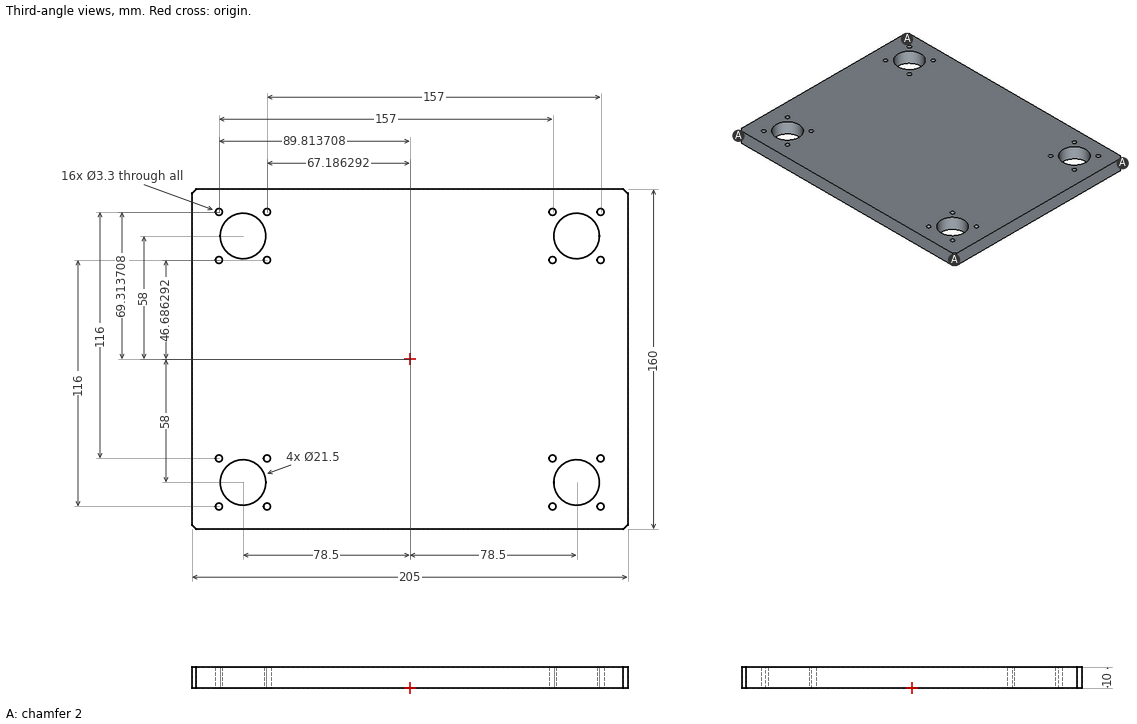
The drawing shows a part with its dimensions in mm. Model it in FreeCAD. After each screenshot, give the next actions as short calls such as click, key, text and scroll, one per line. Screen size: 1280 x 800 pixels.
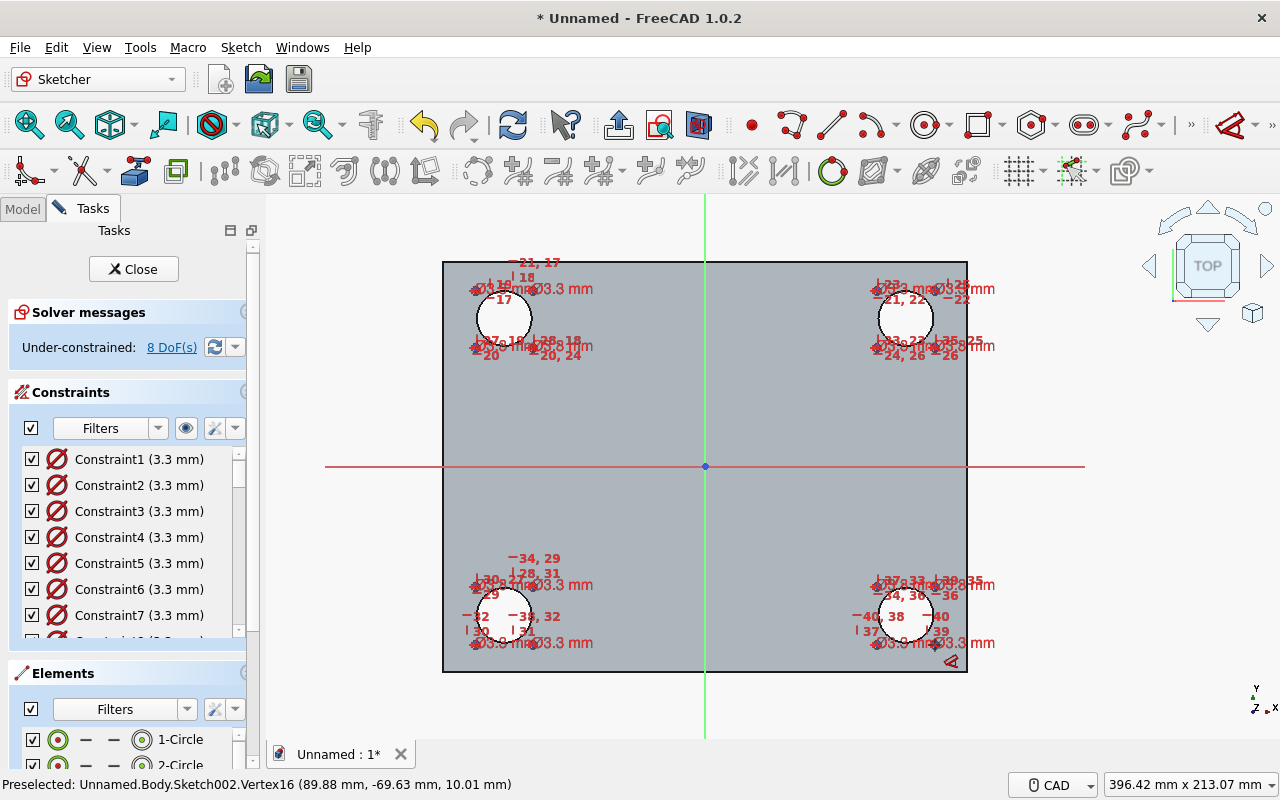
click(476, 291)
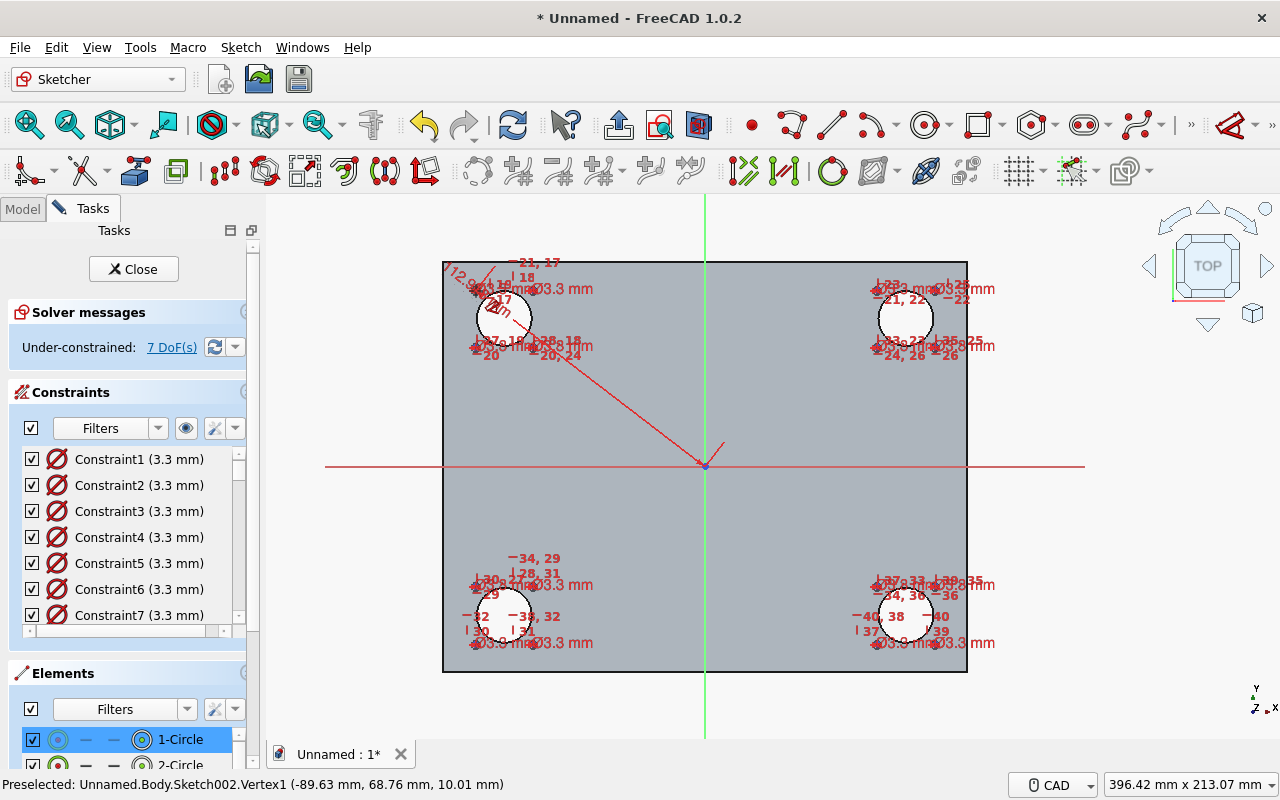
click(877, 291)
click(676, 257)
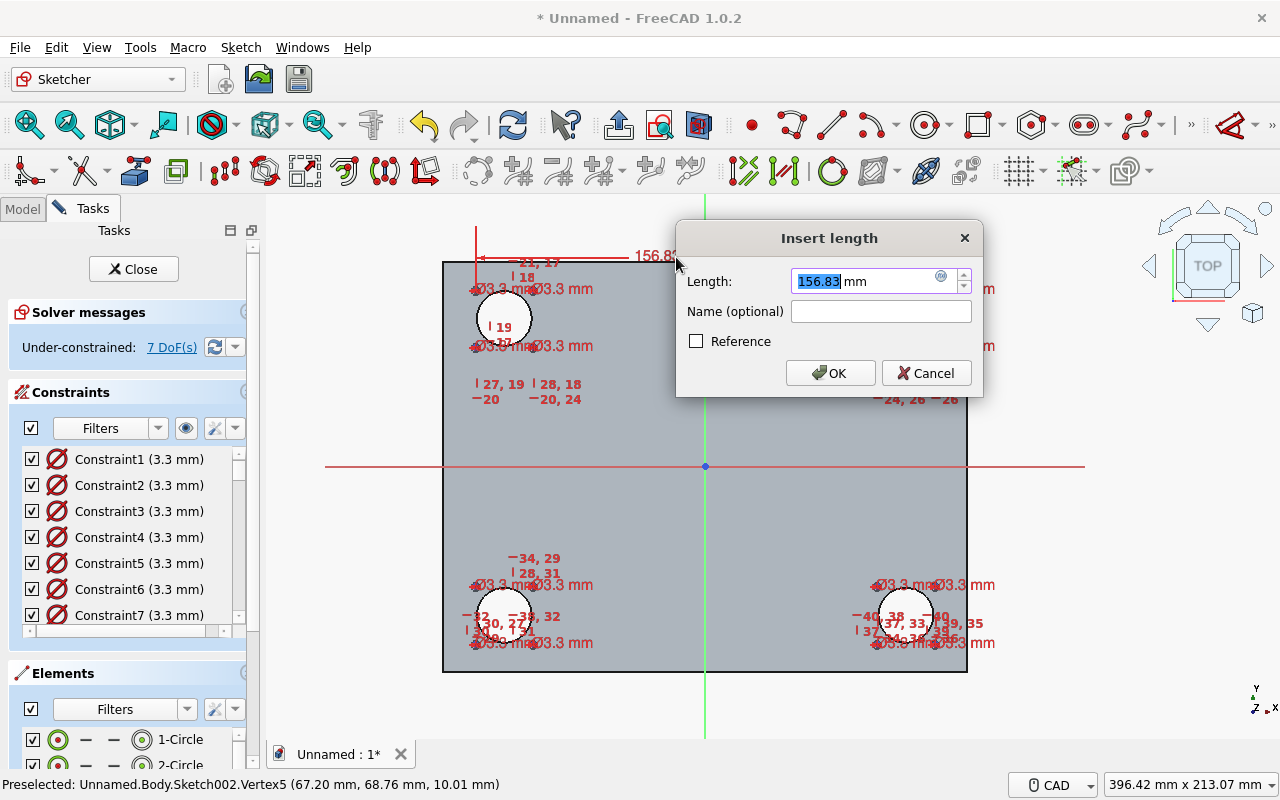
text(157)
key(Return)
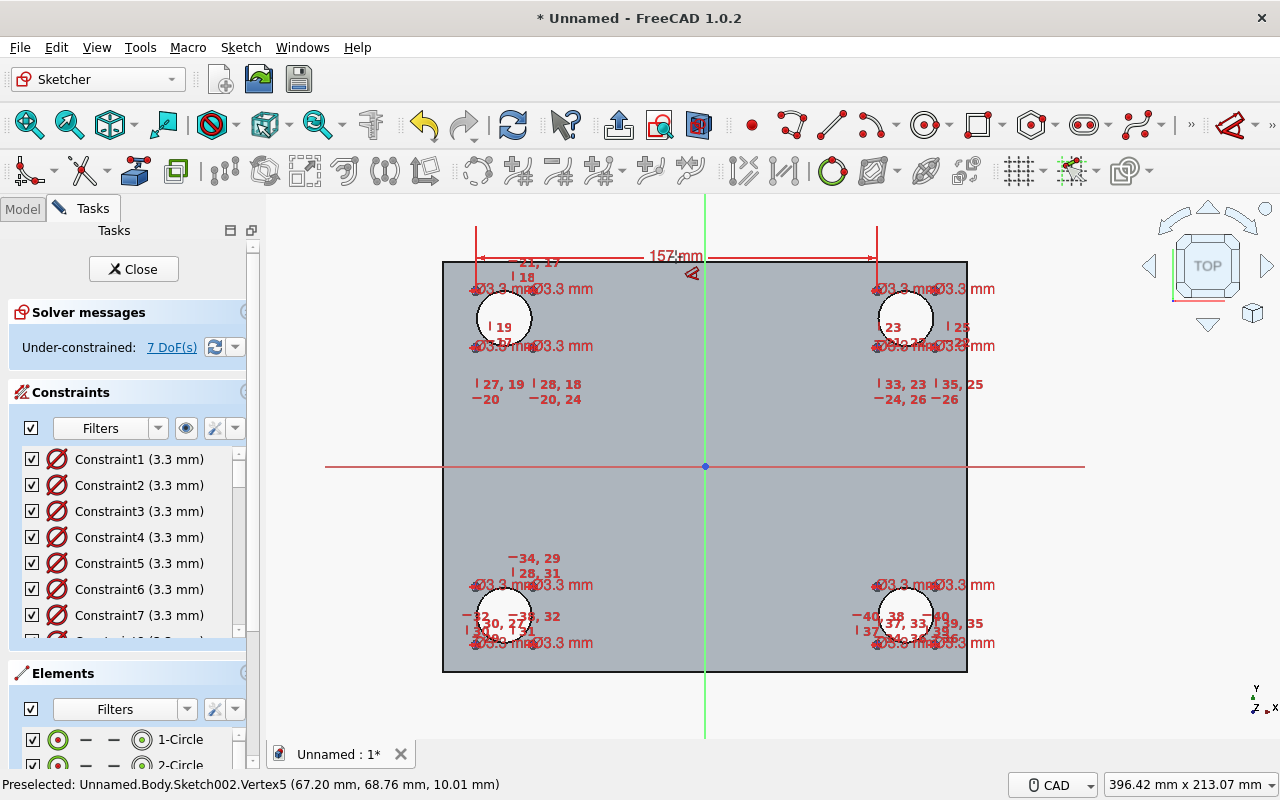
click(533, 291)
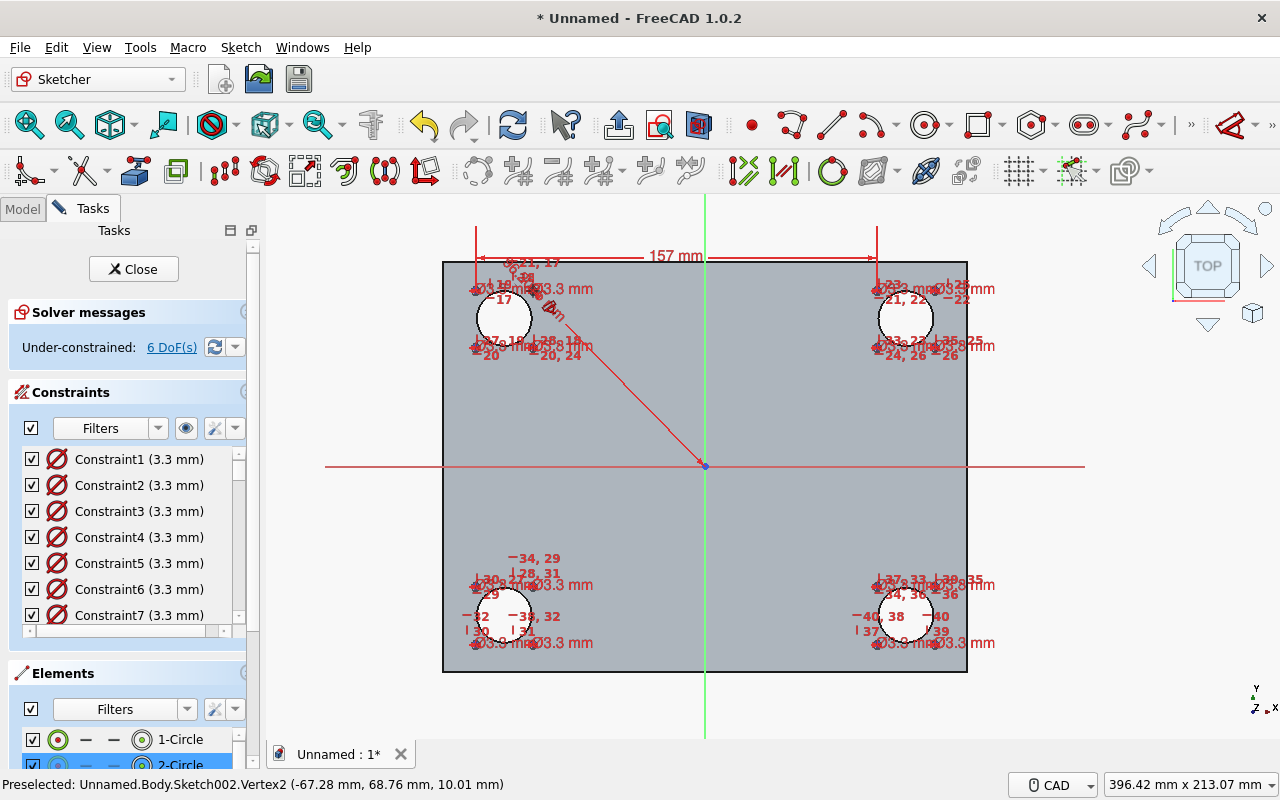
click(935, 291)
click(826, 257)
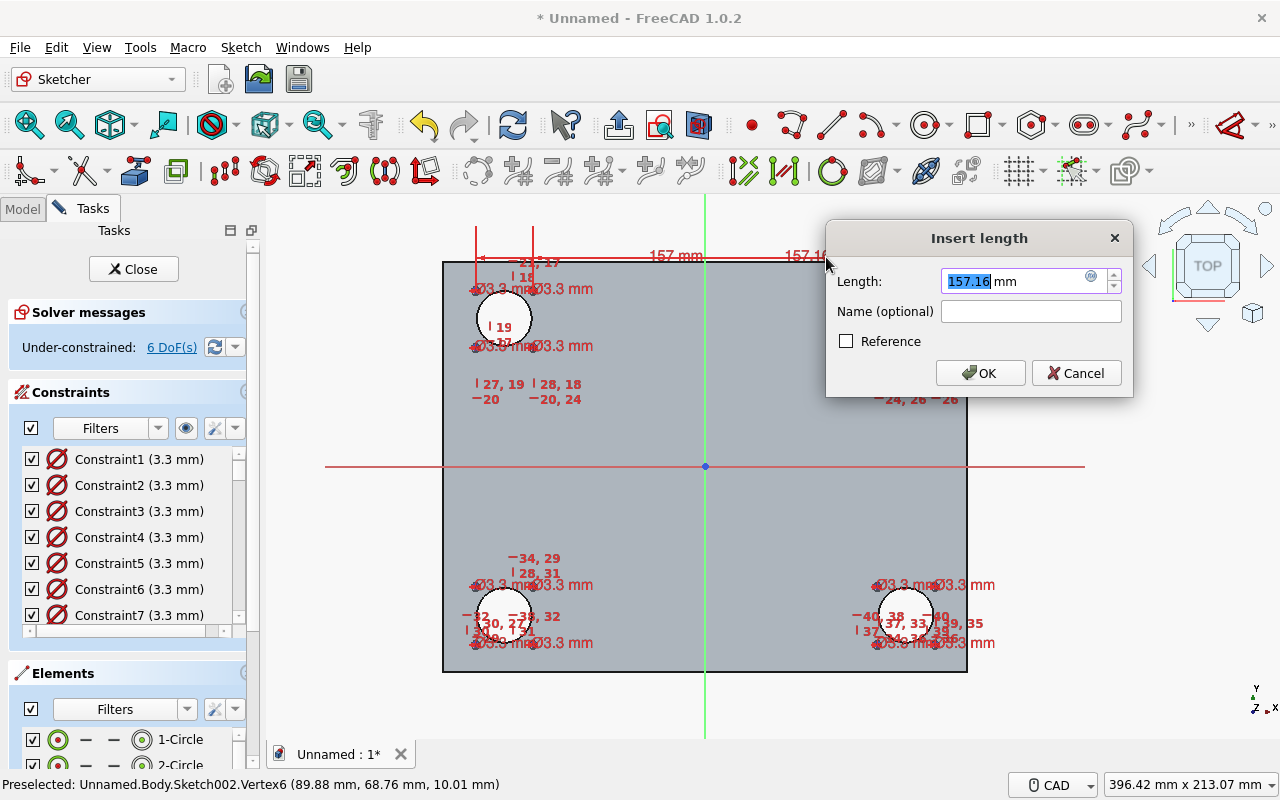
text(157)
key(Return)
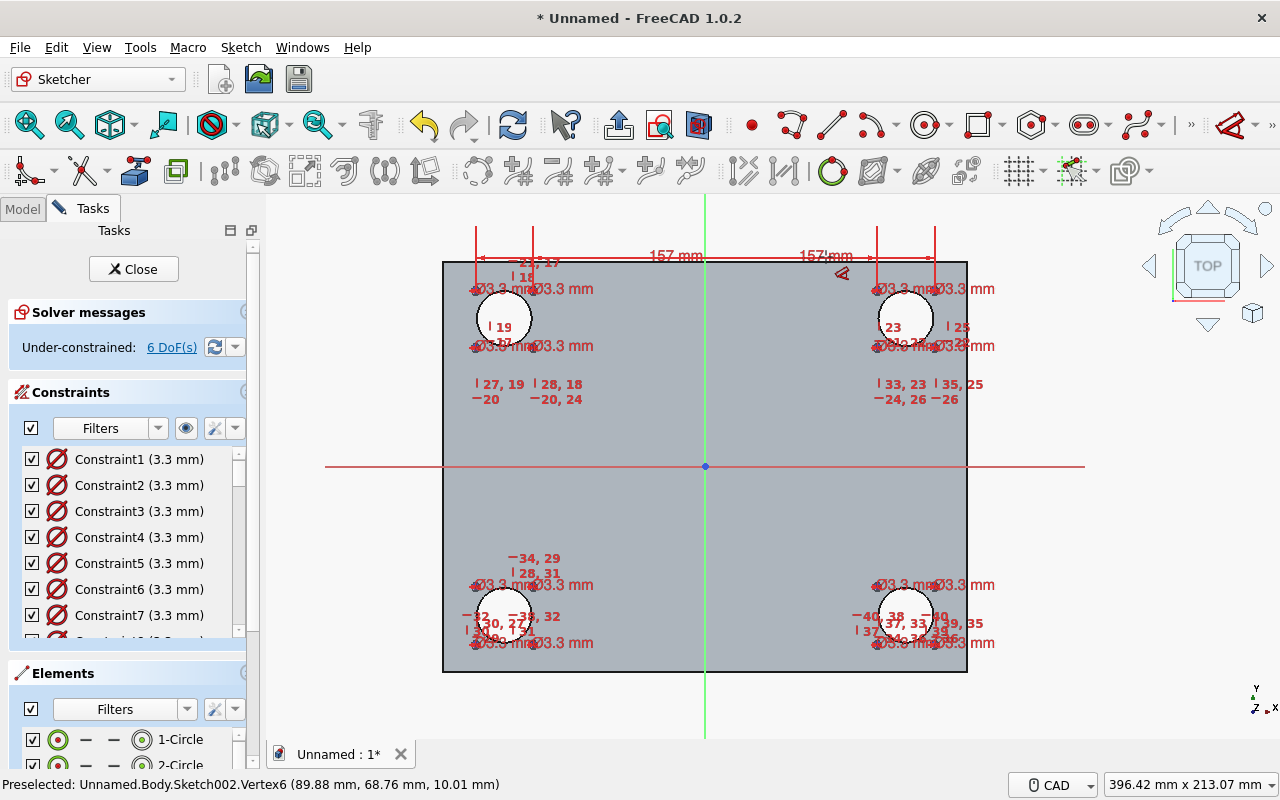
click(476, 291)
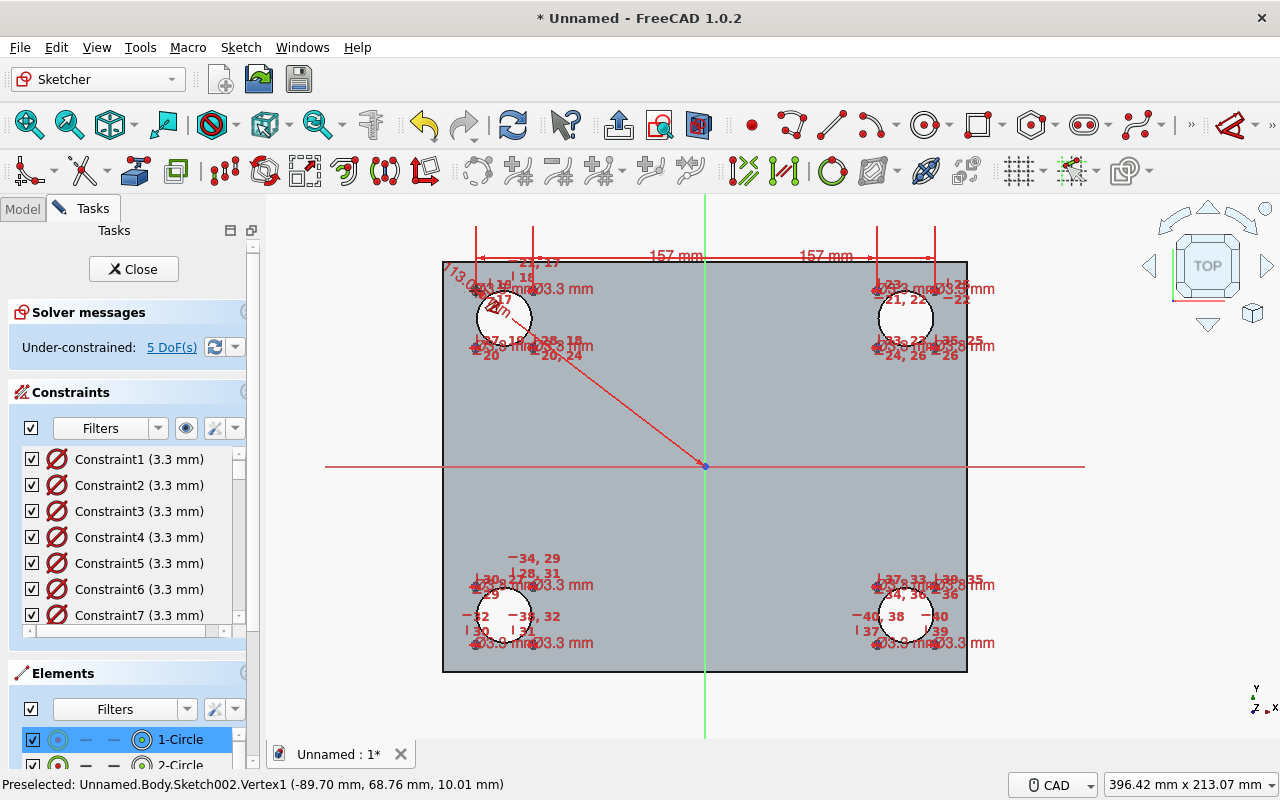
click(476, 587)
click(442, 439)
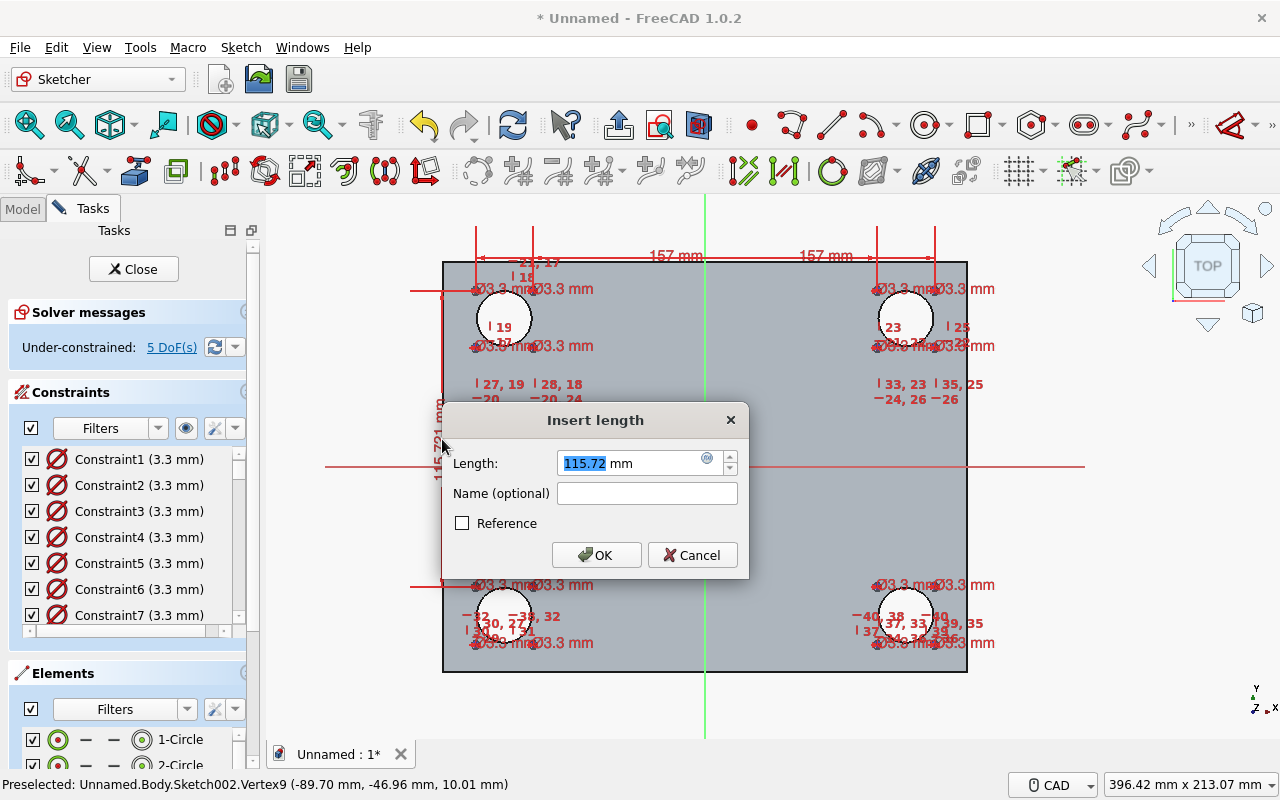
text(116)
key(Return)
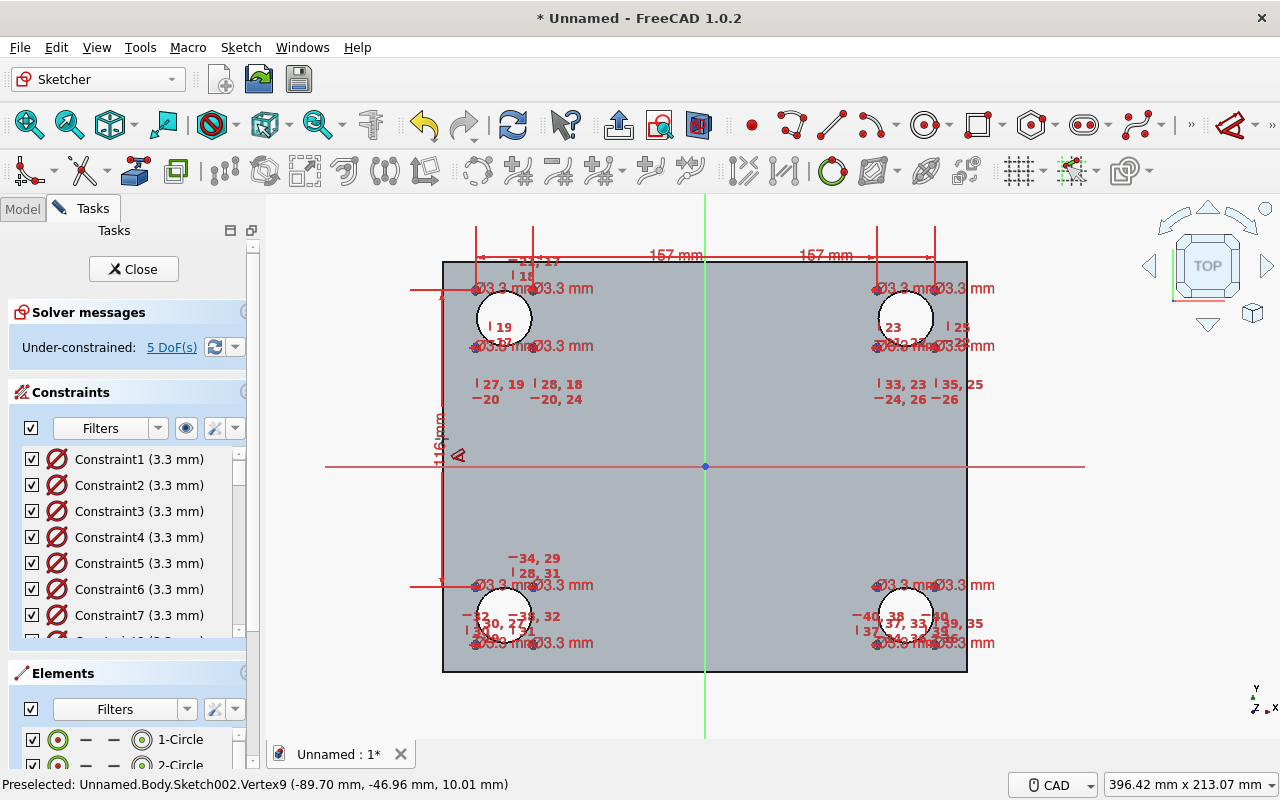
click(476, 348)